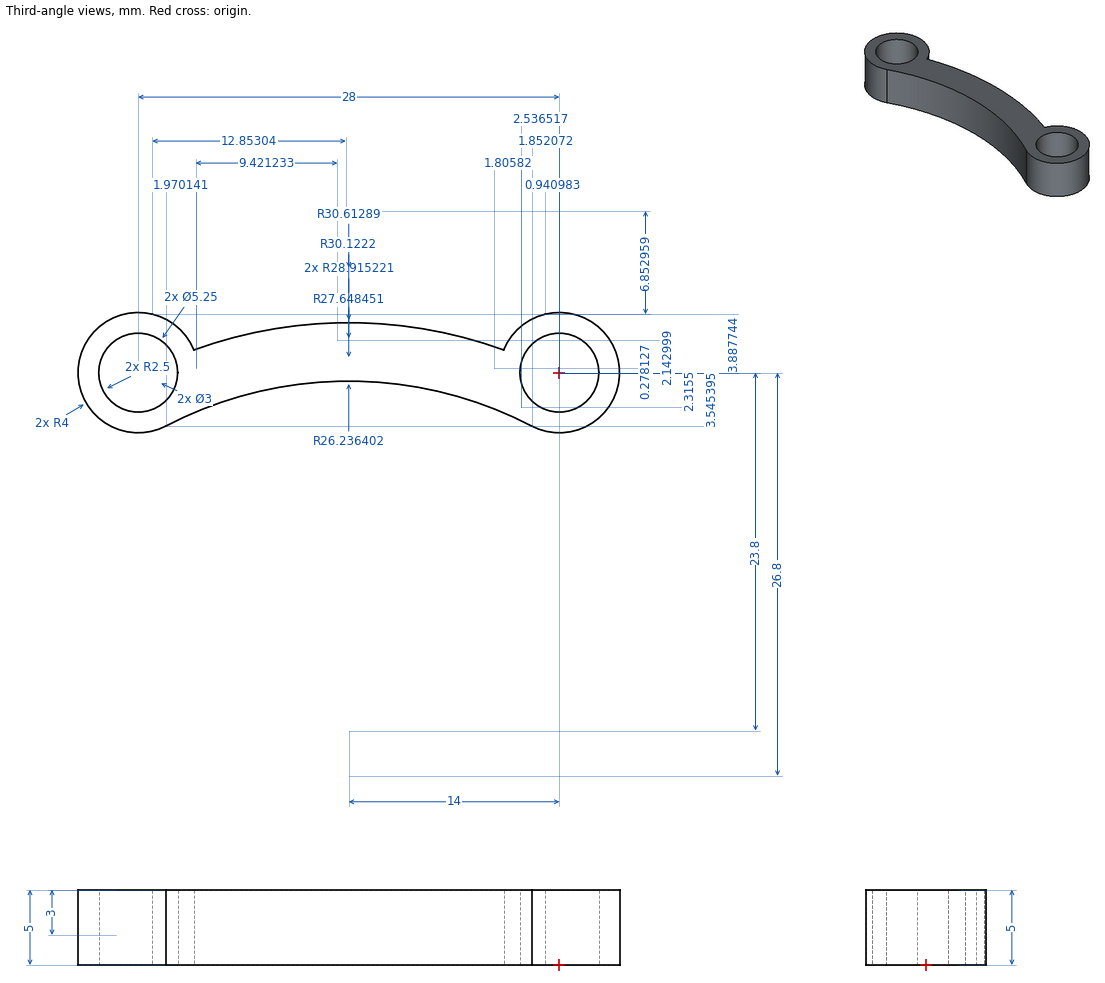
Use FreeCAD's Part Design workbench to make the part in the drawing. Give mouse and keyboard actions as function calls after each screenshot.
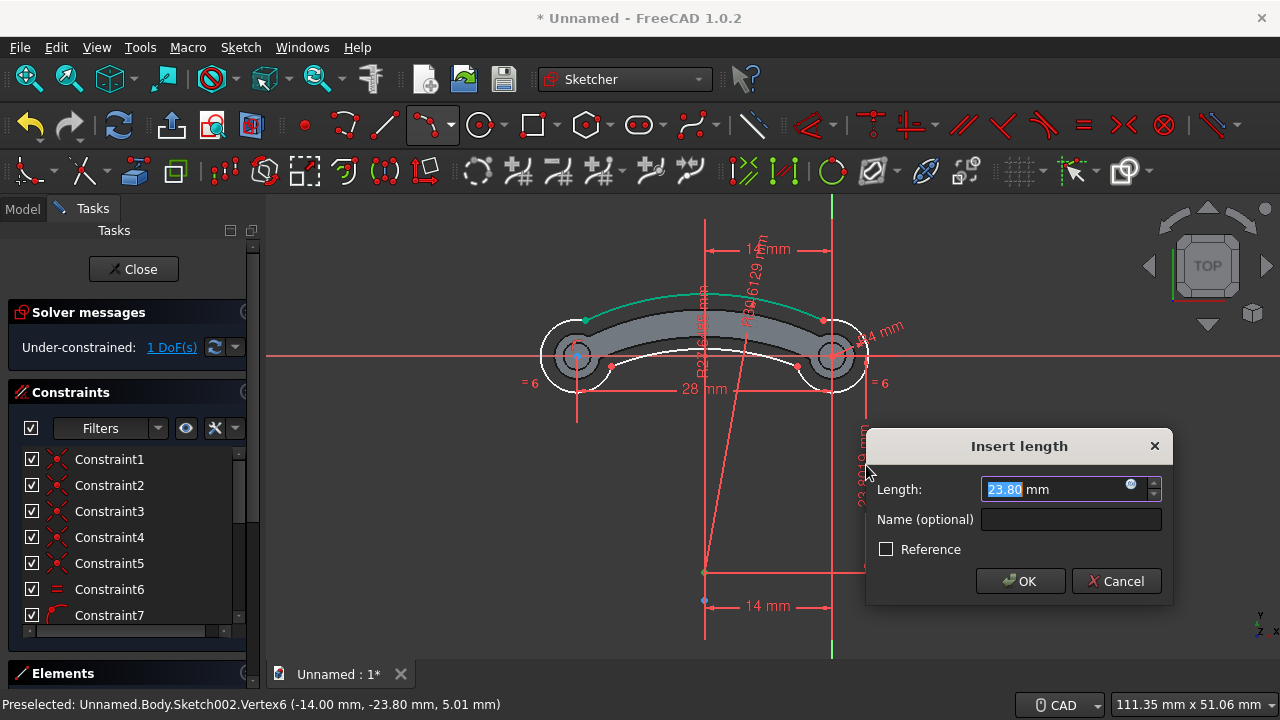
text(23.8)
key(Return)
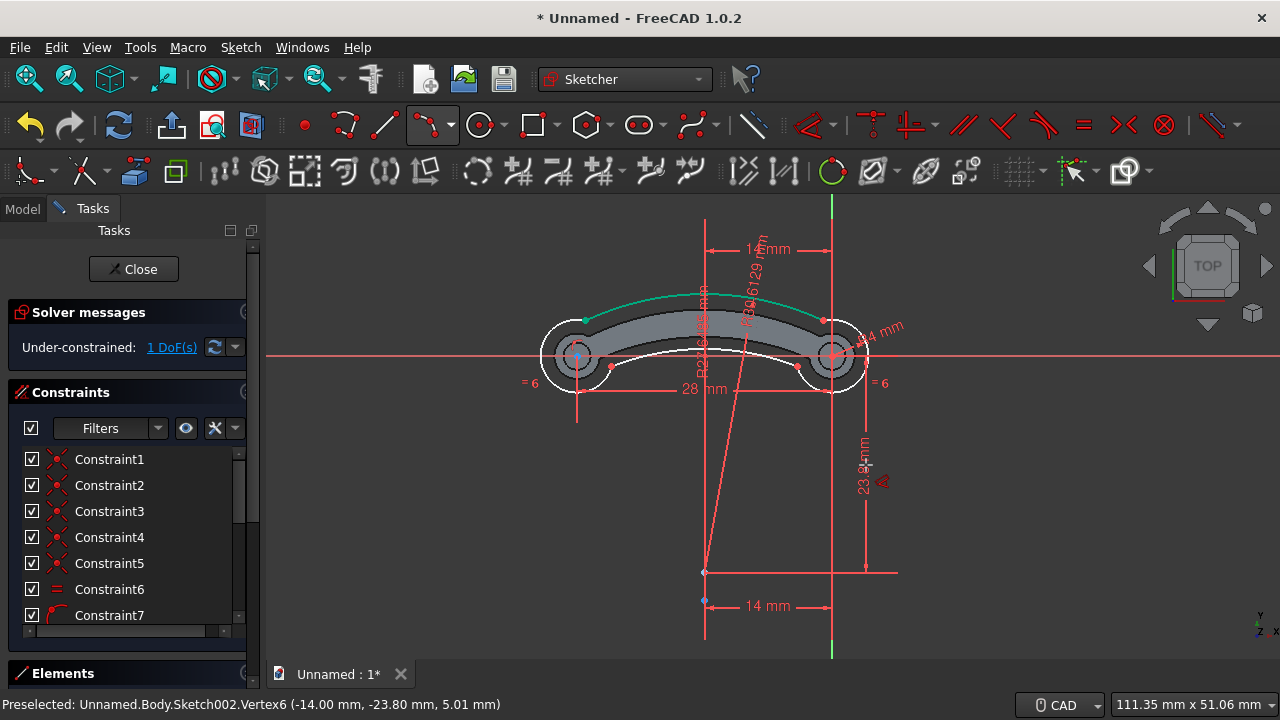
click(705, 601)
click(866, 422)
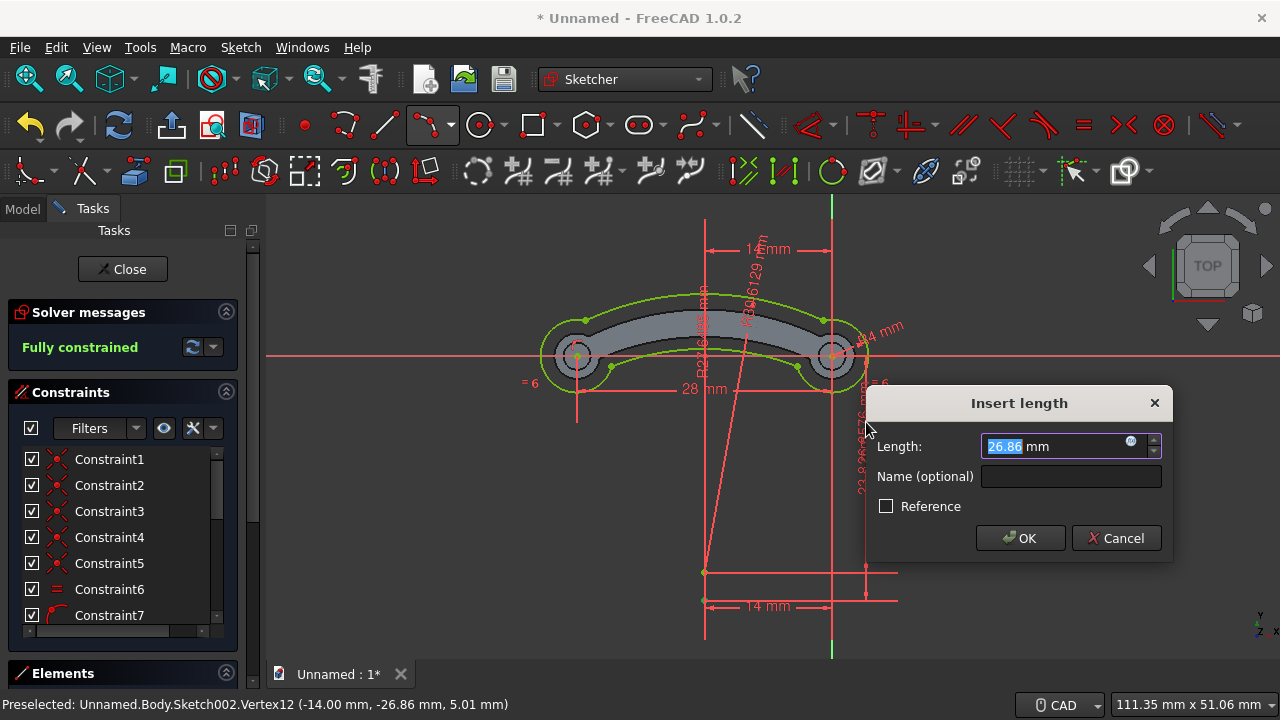
text(26.8)
key(Return)
key(Escape)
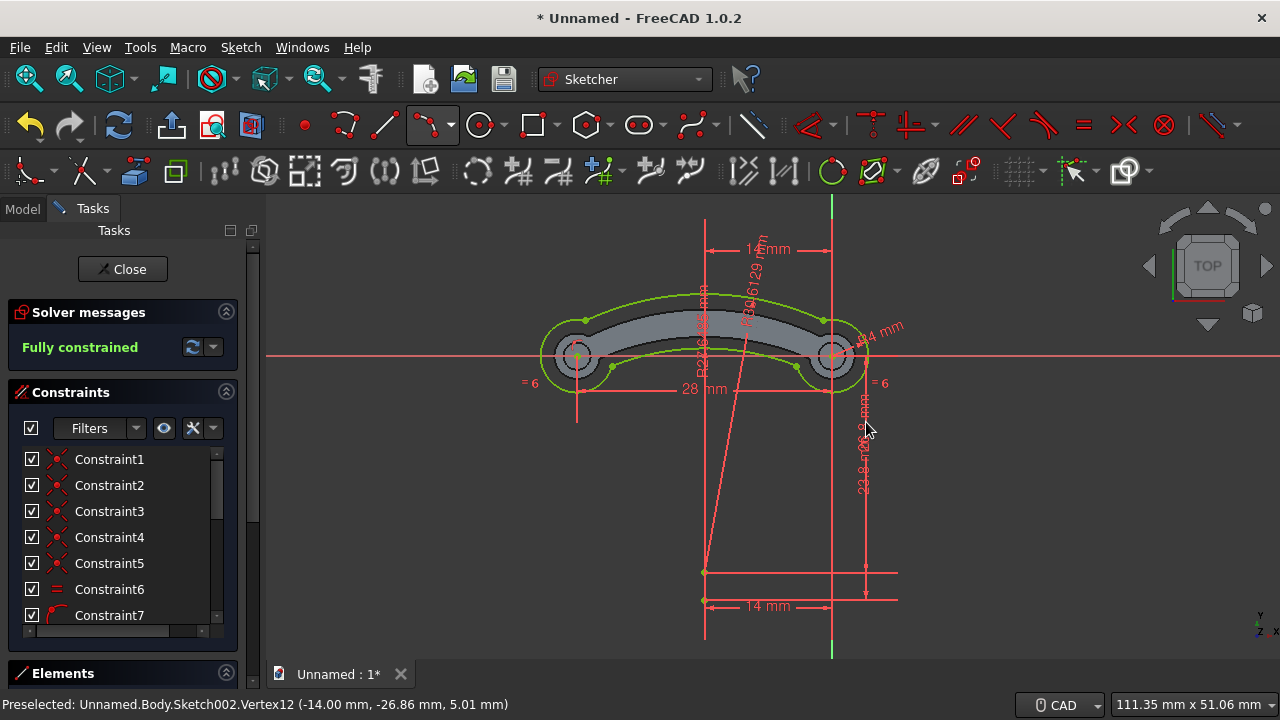
click(123, 269)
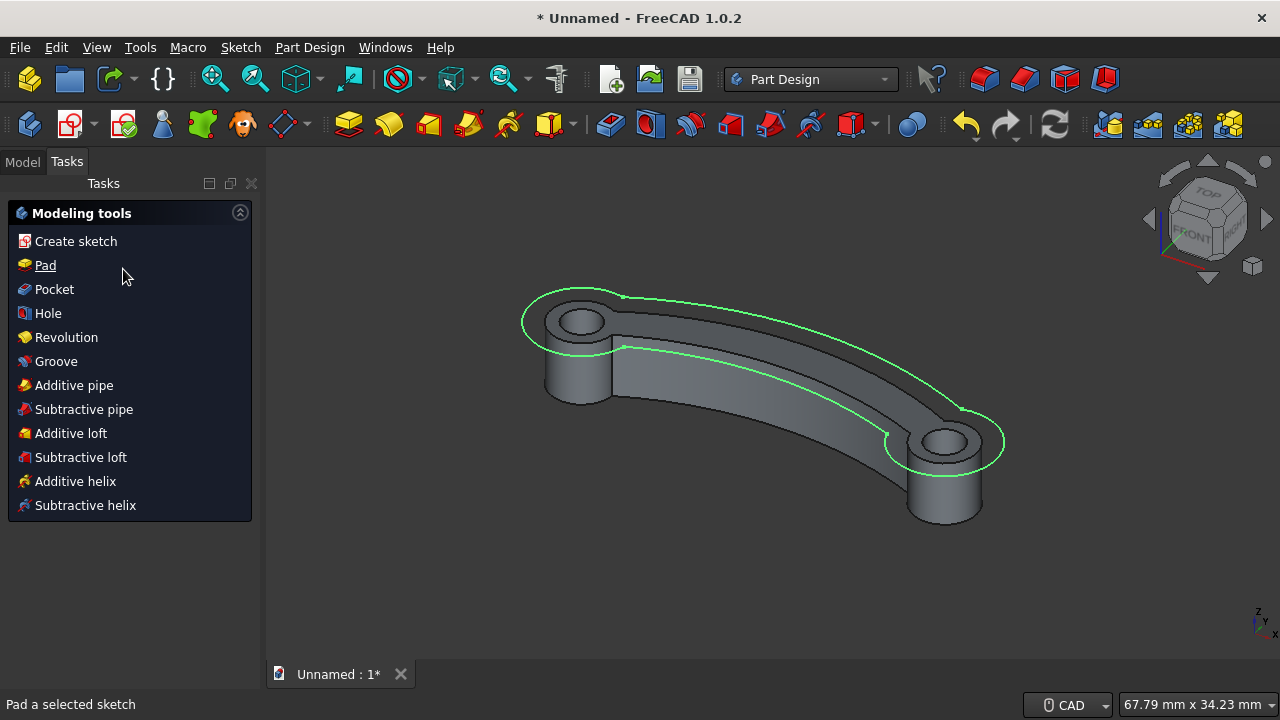
click(350, 124)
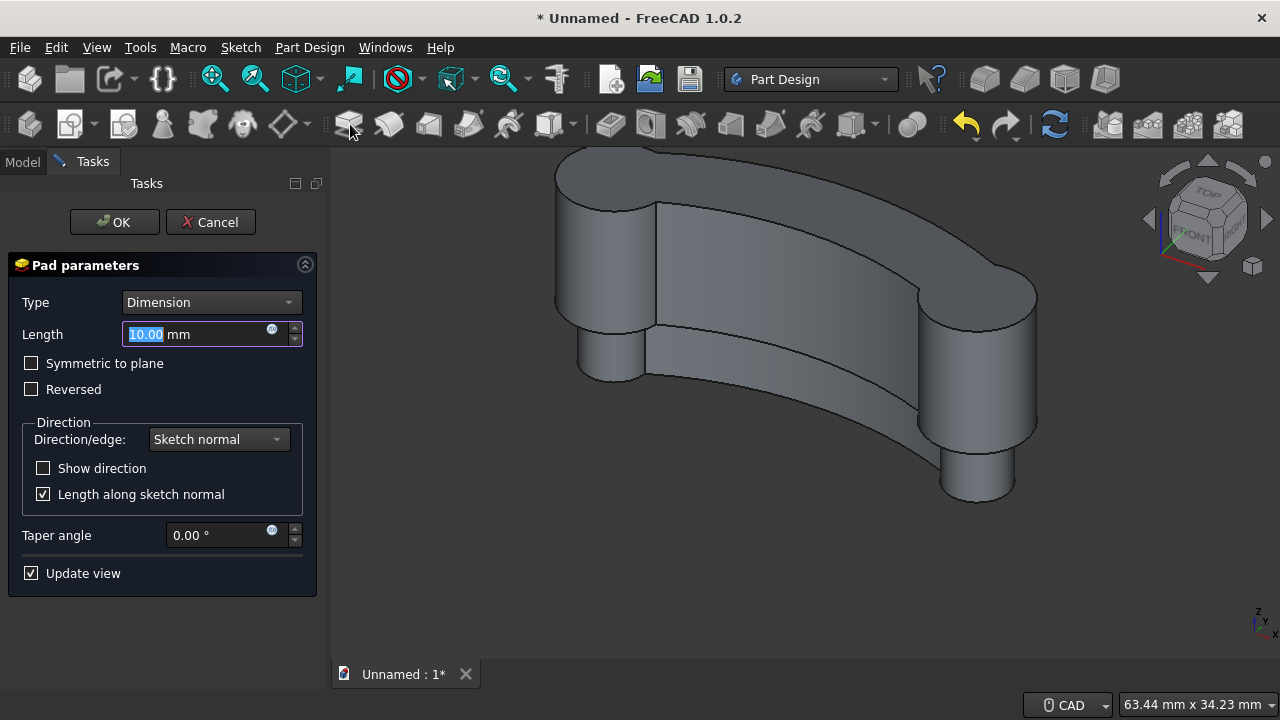
text(5)
key(Tab)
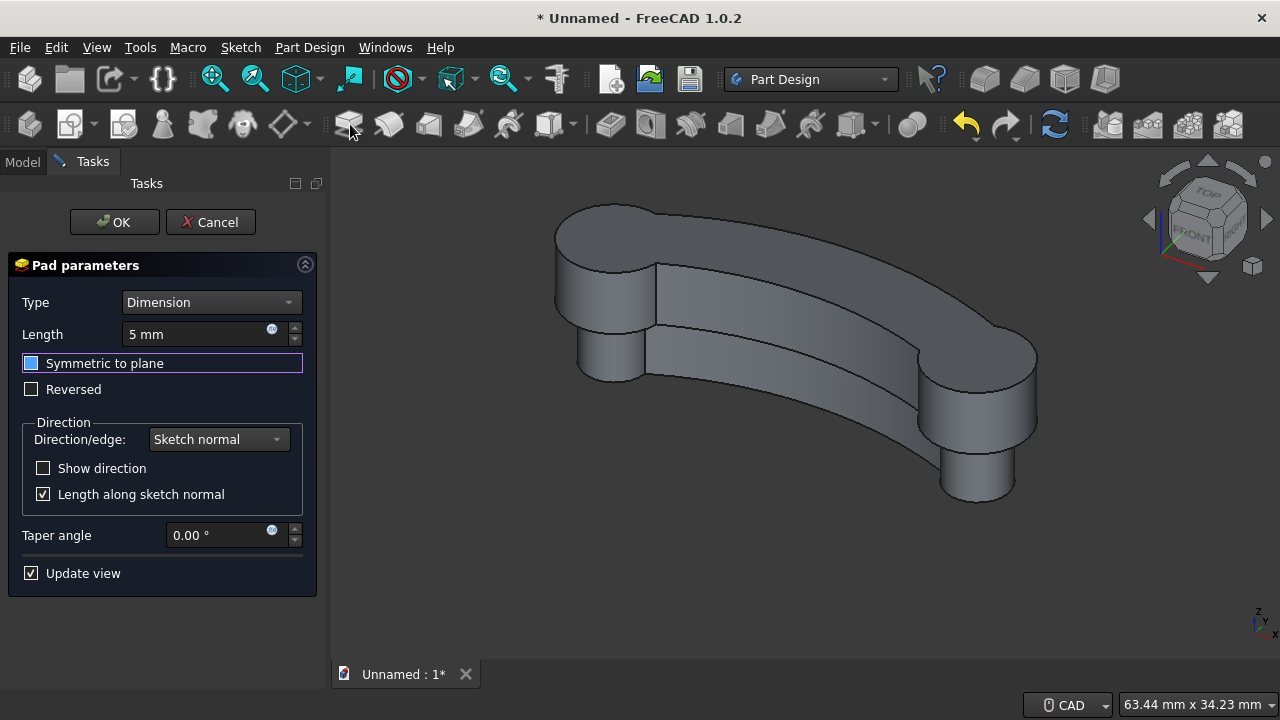
click(30, 389)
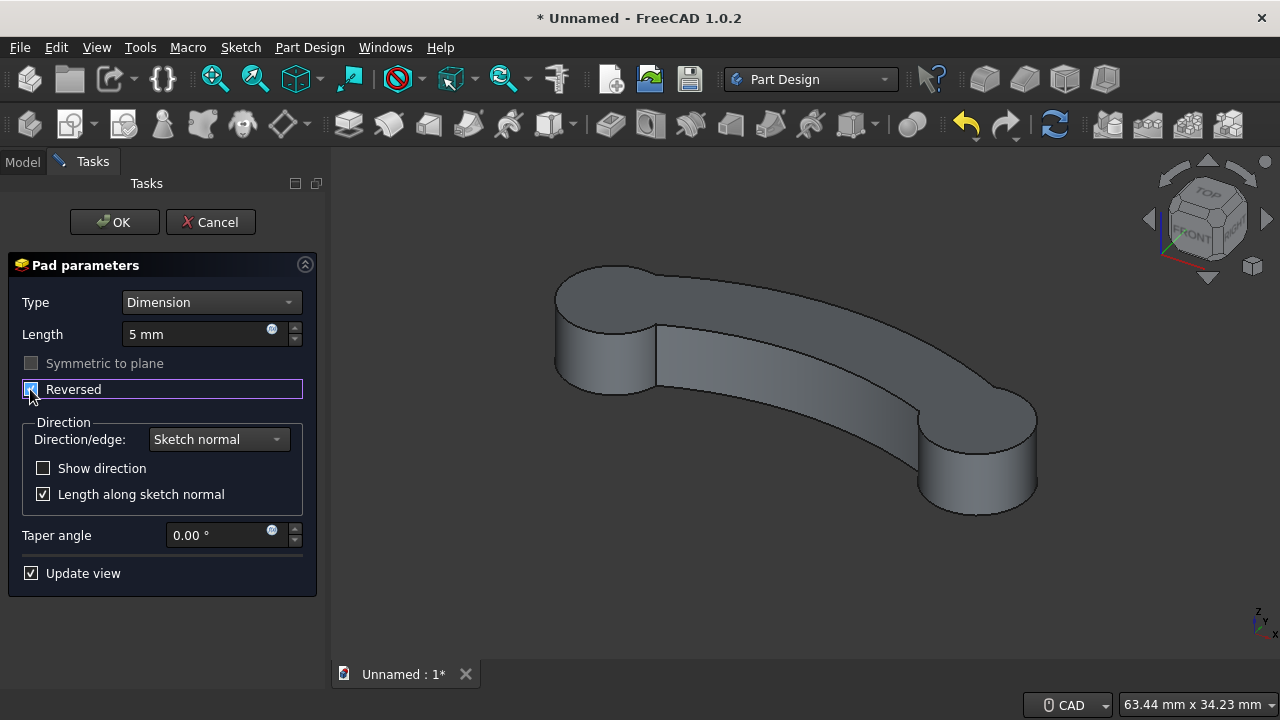
click(115, 222)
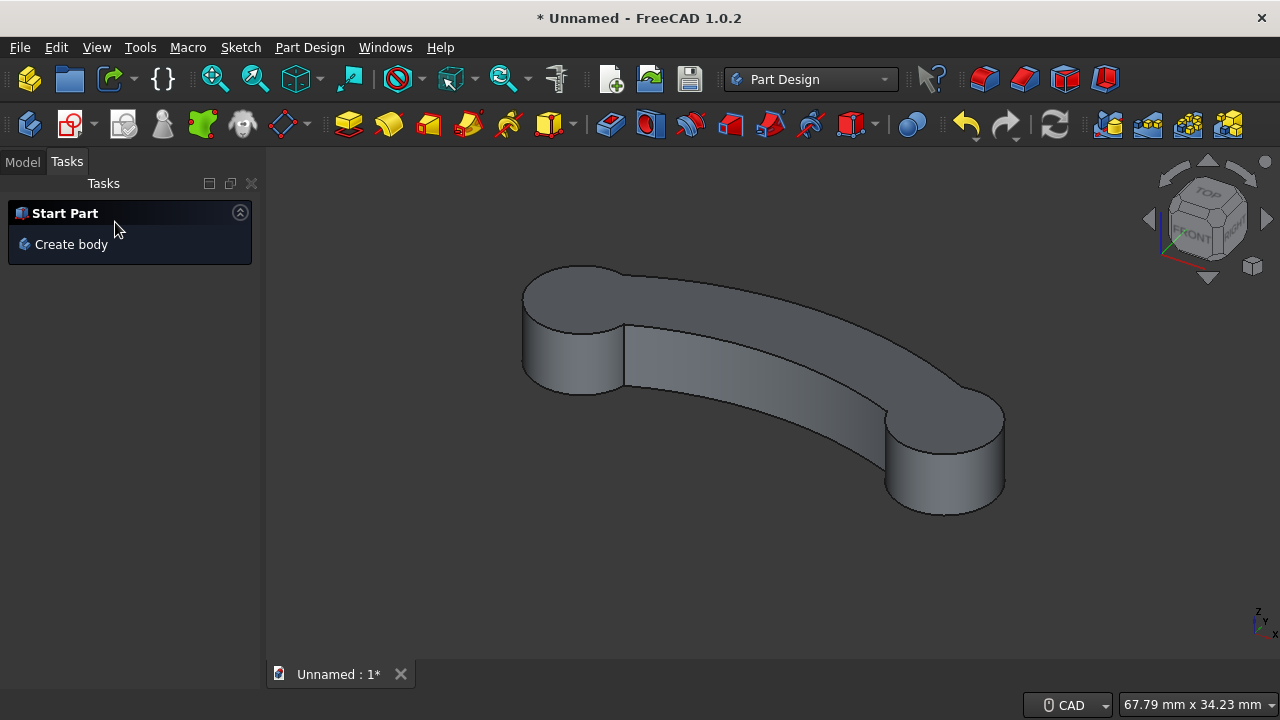
click(962, 426)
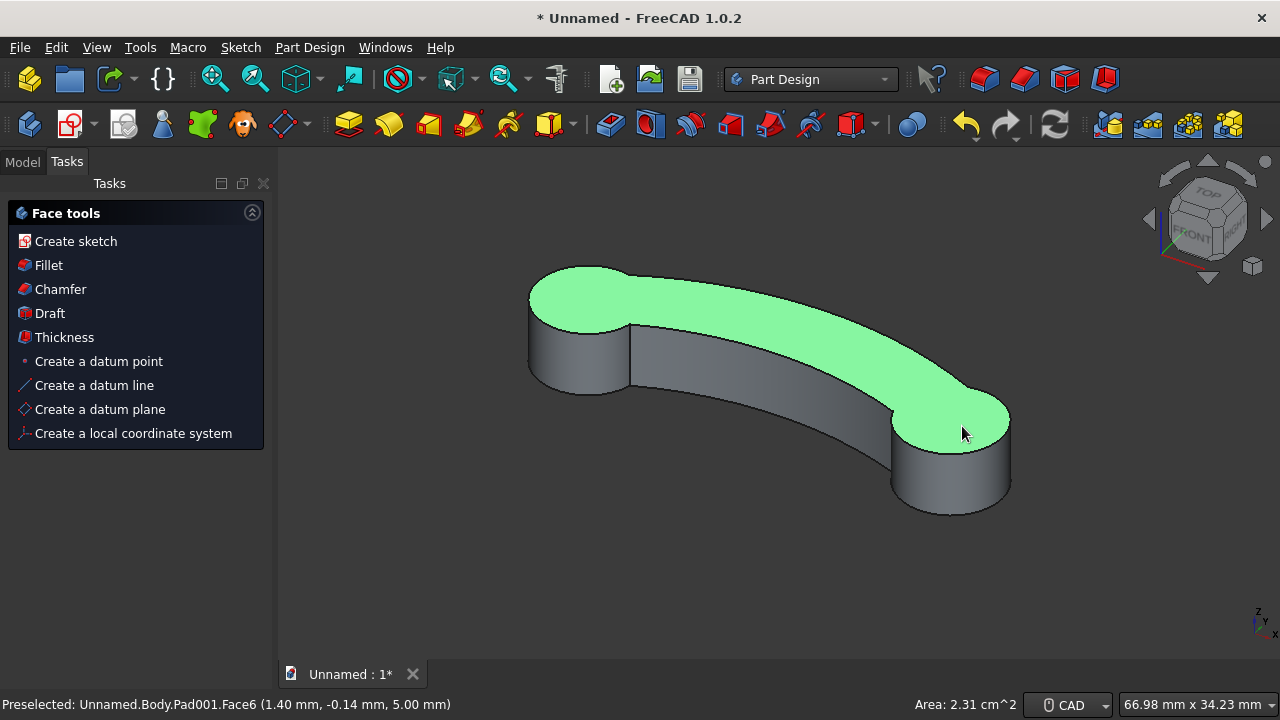
click(70, 124)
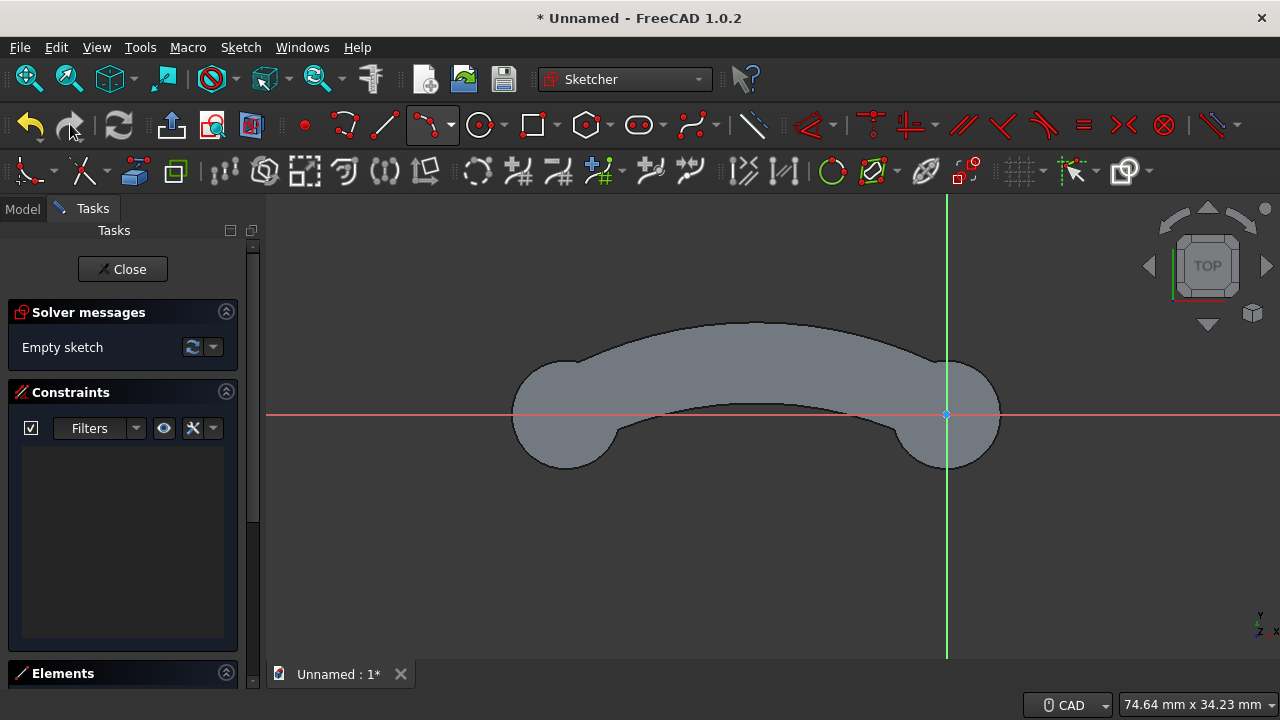
click(480, 126)